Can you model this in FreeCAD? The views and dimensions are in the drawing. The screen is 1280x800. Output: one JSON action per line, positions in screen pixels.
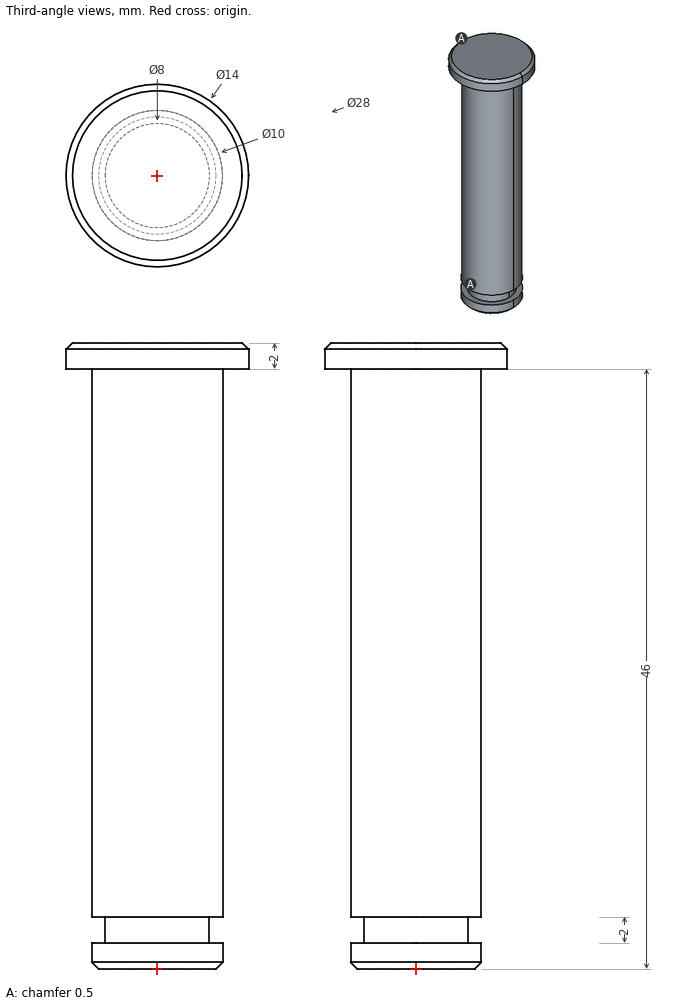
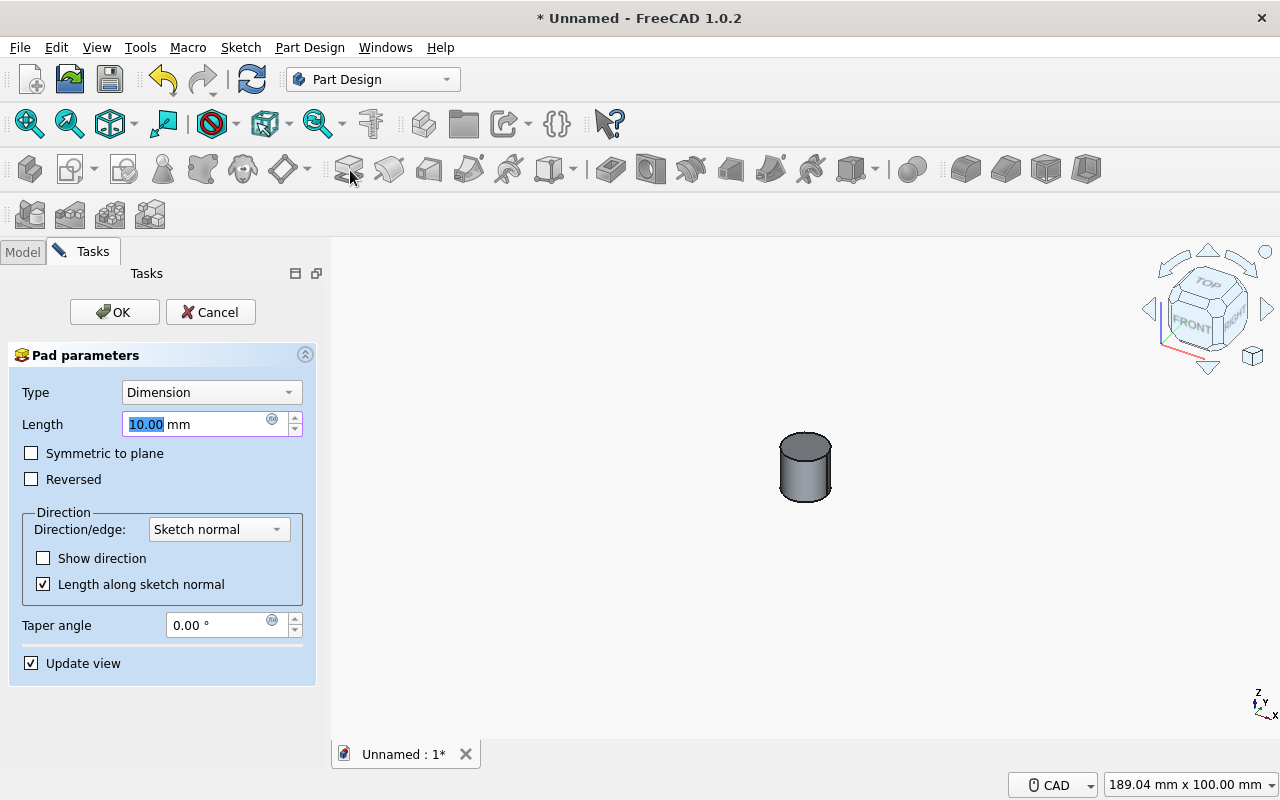
{"action": "type", "text": "46"}
{"action": "key", "text": "Tab"}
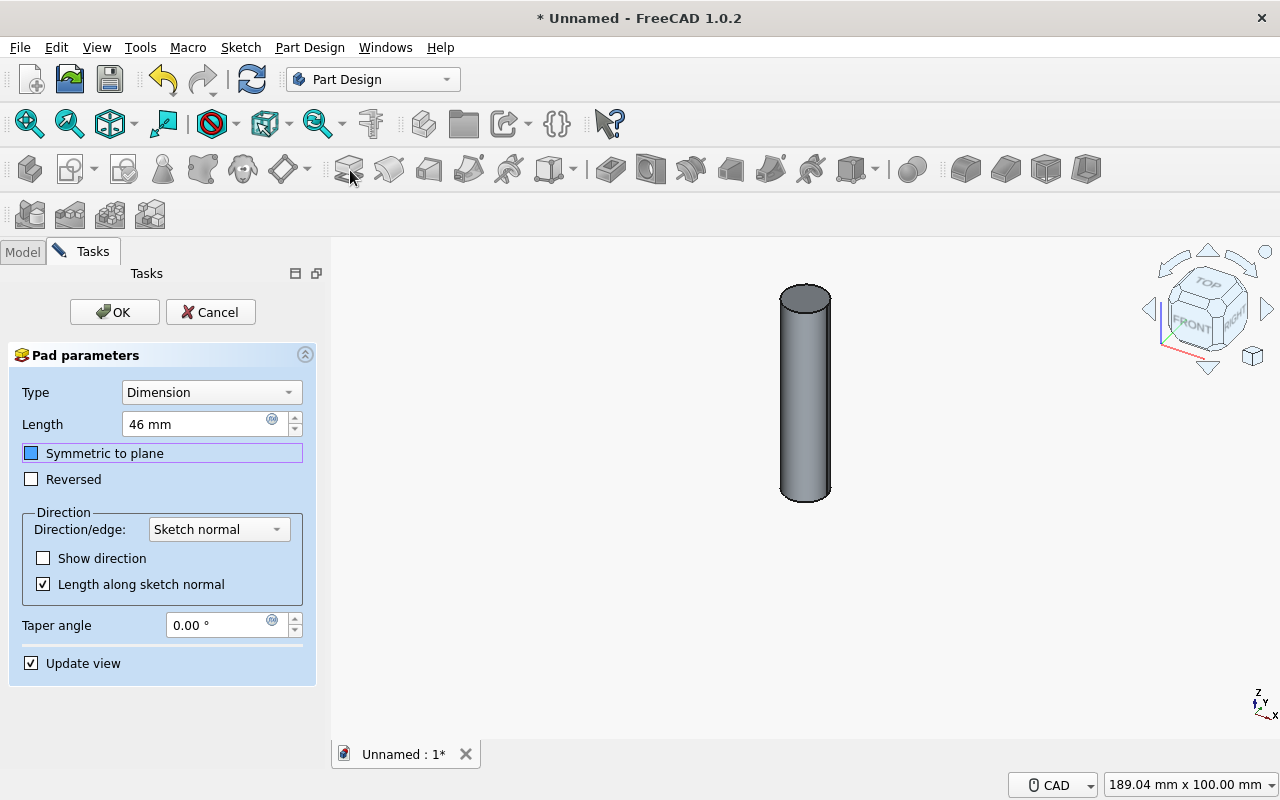
{"action": "left_click", "coordinate": [115, 312]}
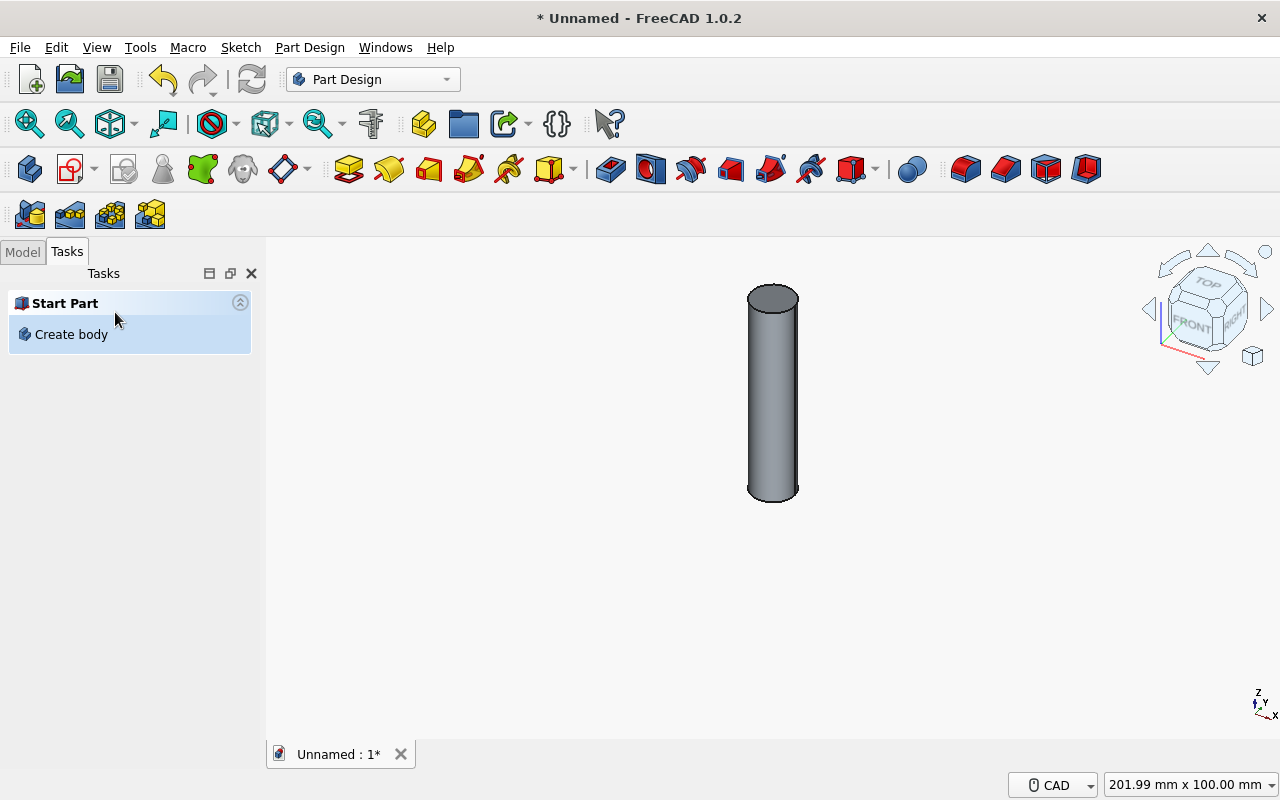
{"action": "left_click", "coordinate": [773, 298]}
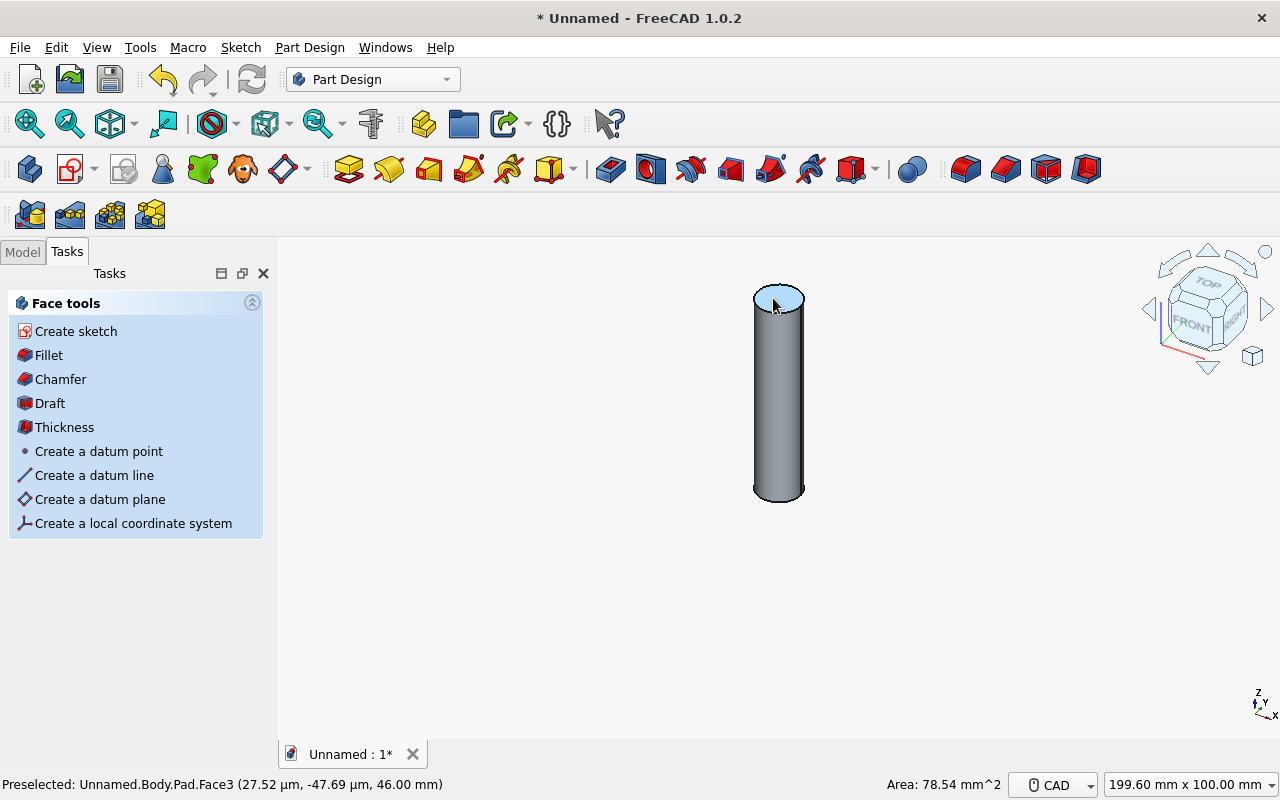
{"action": "left_click", "coordinate": [70, 170]}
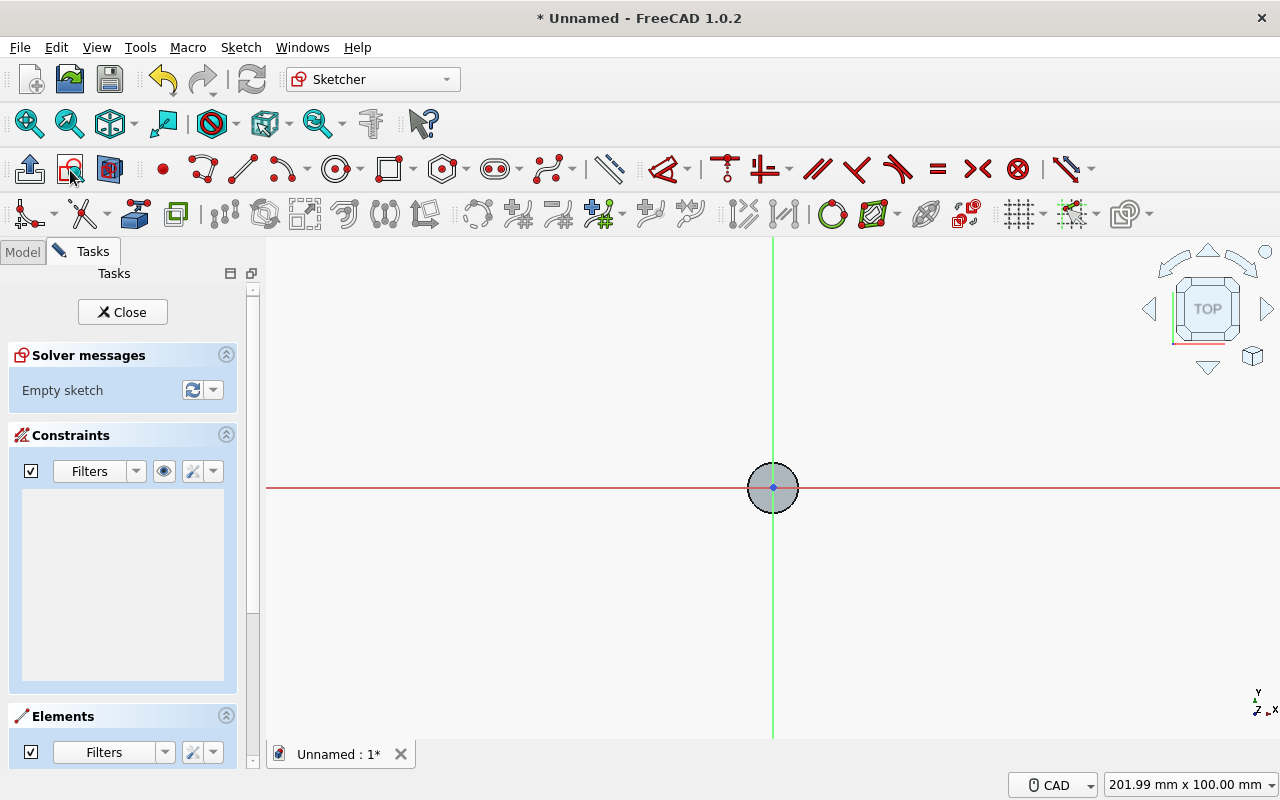
{"action": "scroll", "coordinate": [795, 488], "scroll_direction": "up", "scroll_amount": 7}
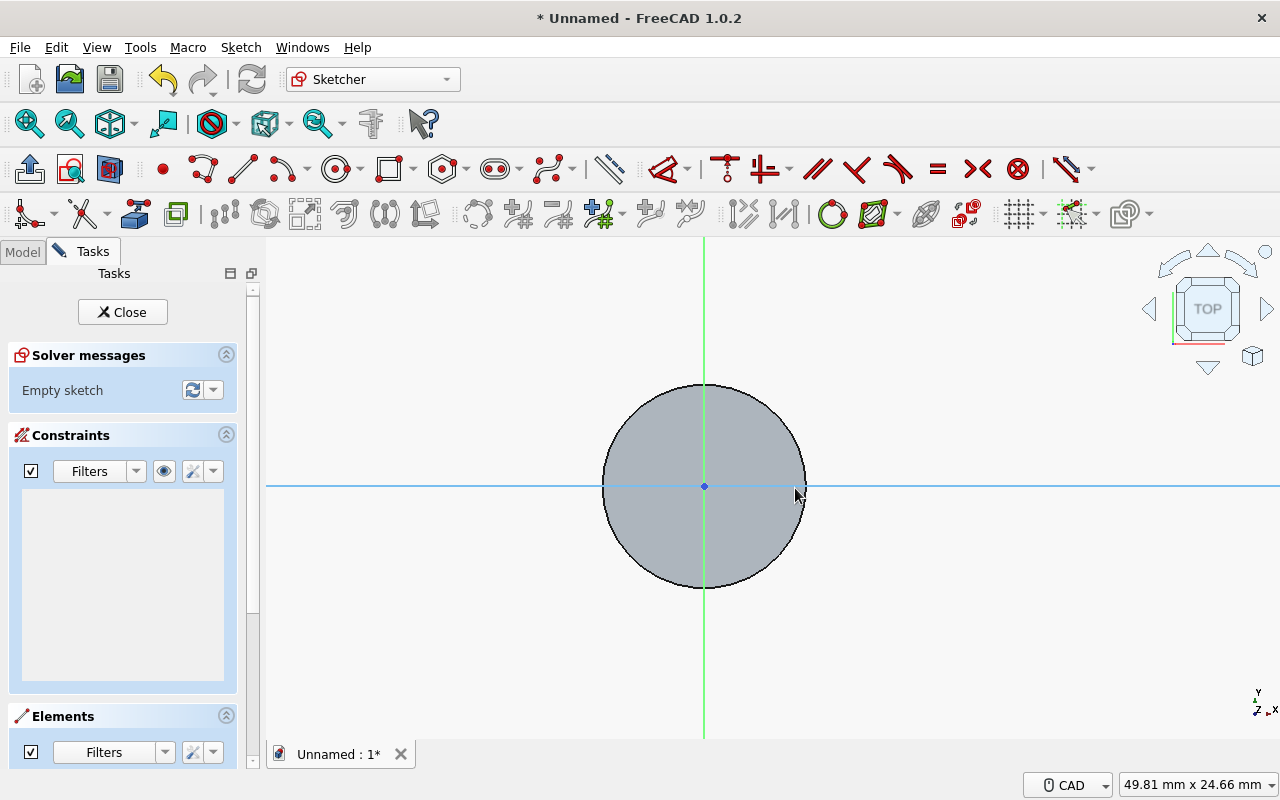
{"action": "key", "text": "g c"}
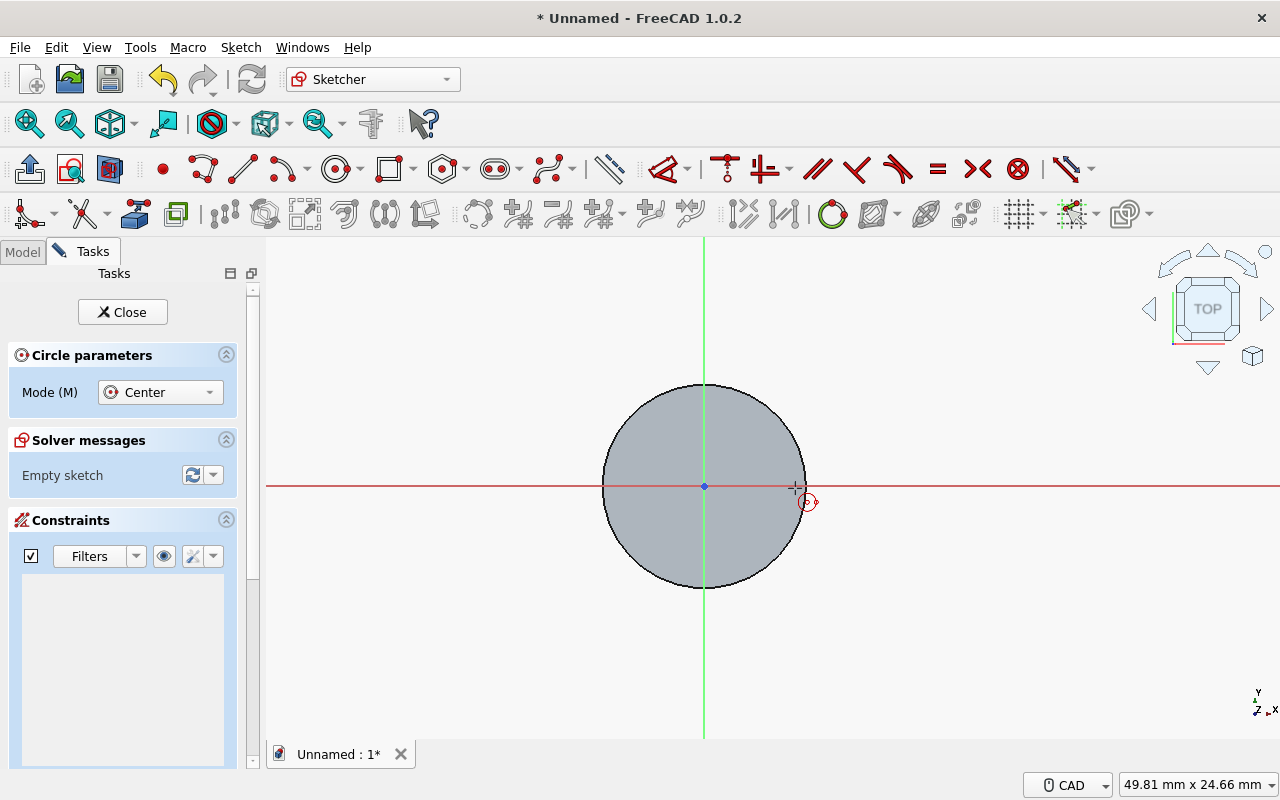
{"action": "left_click", "coordinate": [704, 486]}
{"action": "mouse_move", "coordinate": [805, 386]}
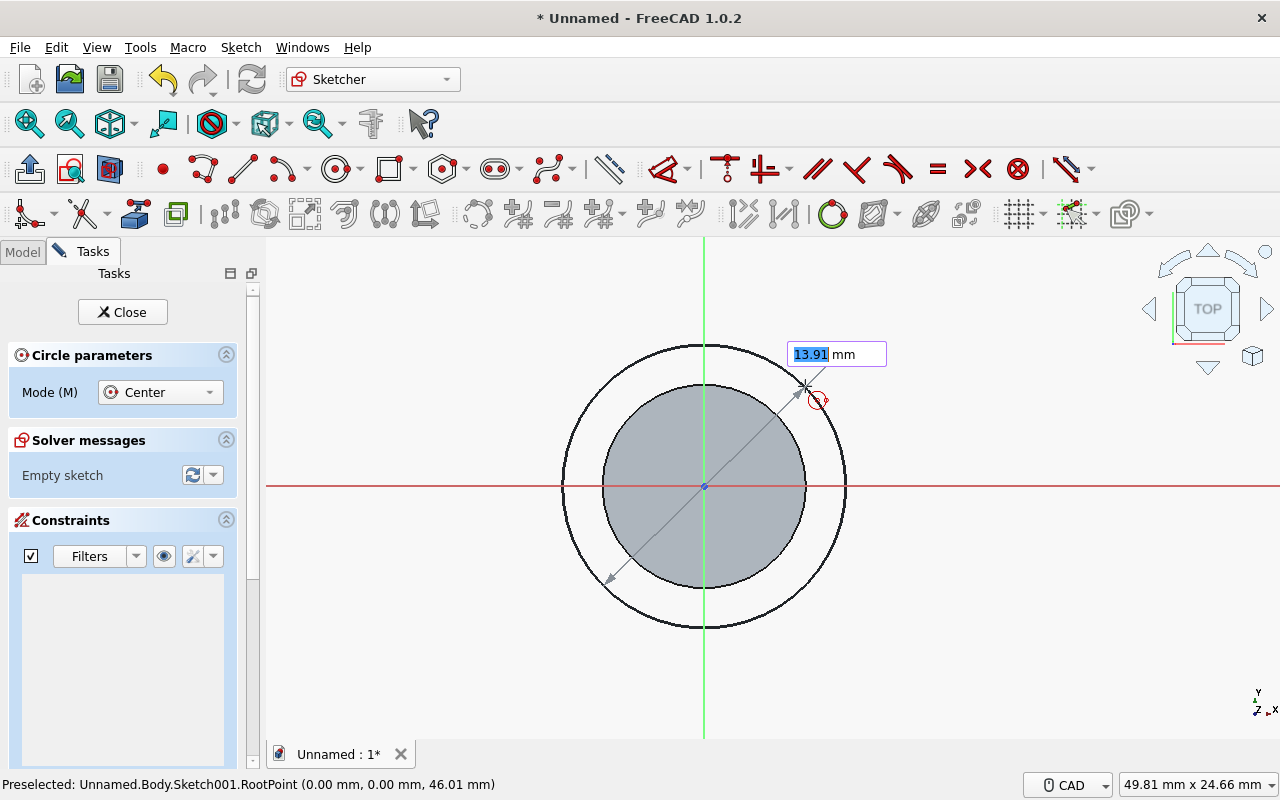
{"action": "type", "text": "14"}
{"action": "key", "text": "Return"}
{"action": "key", "text": "Escape"}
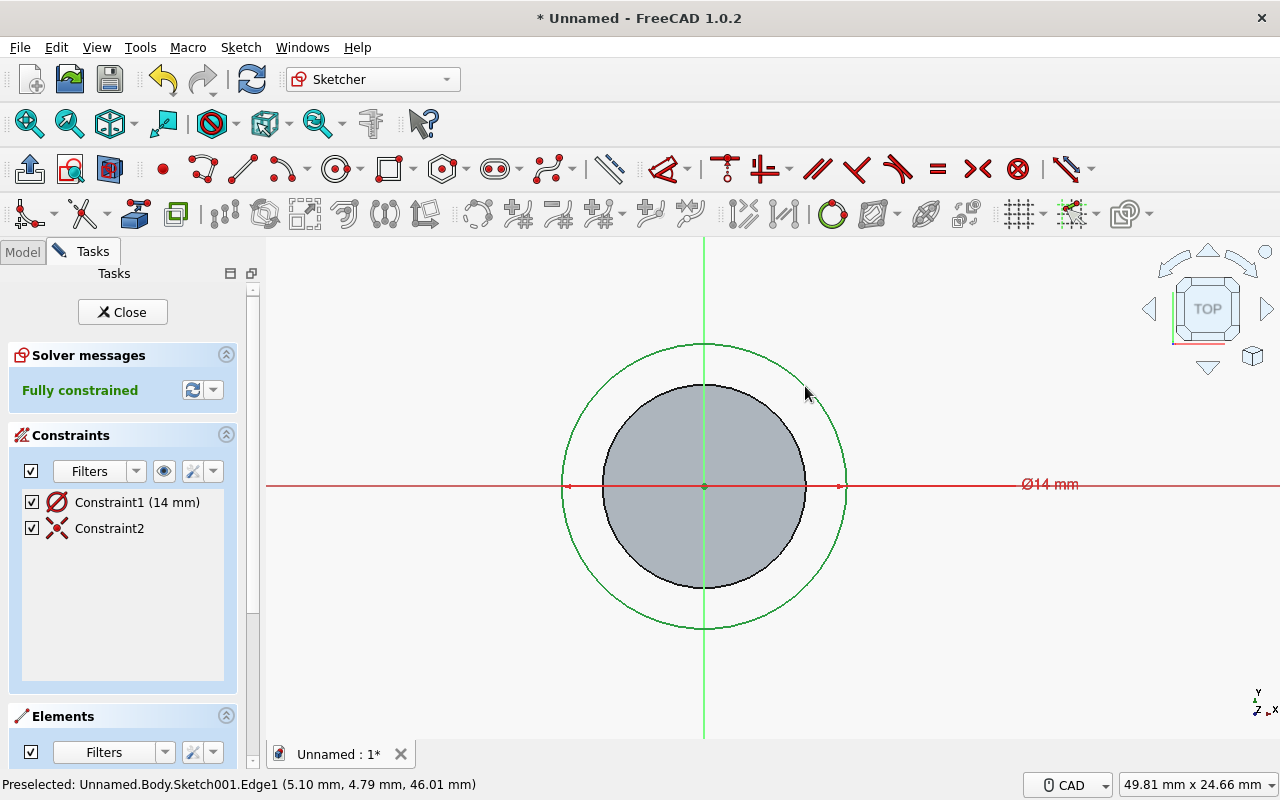
{"action": "left_click", "coordinate": [123, 312]}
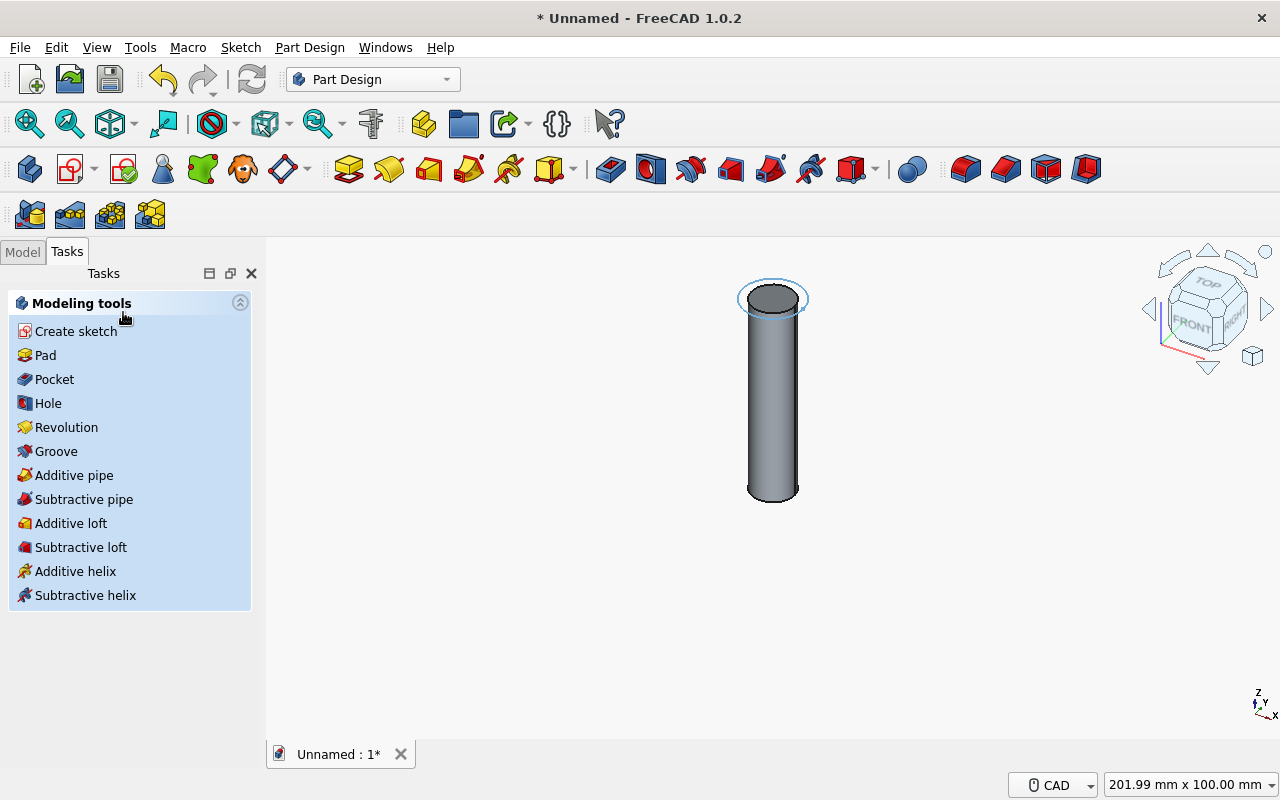
{"action": "left_click", "coordinate": [350, 170]}